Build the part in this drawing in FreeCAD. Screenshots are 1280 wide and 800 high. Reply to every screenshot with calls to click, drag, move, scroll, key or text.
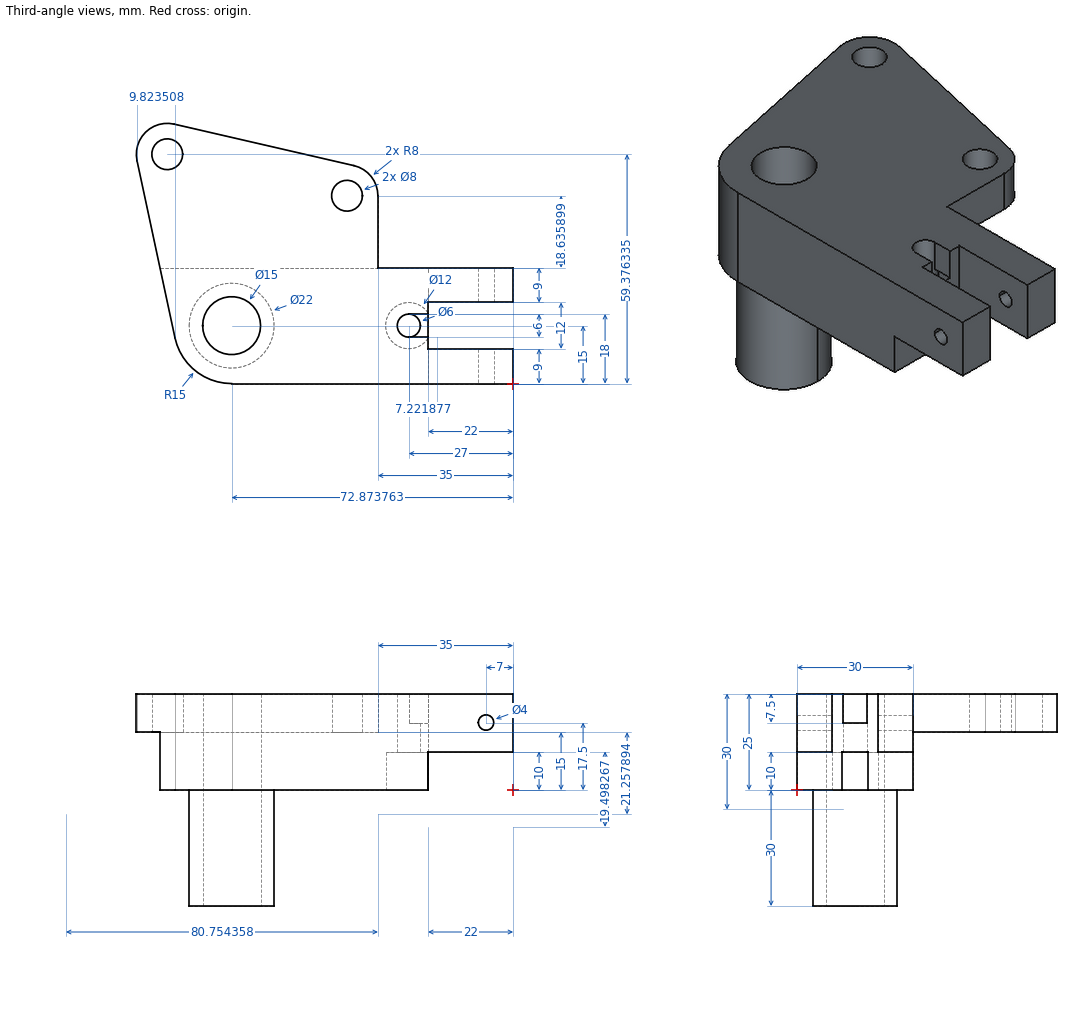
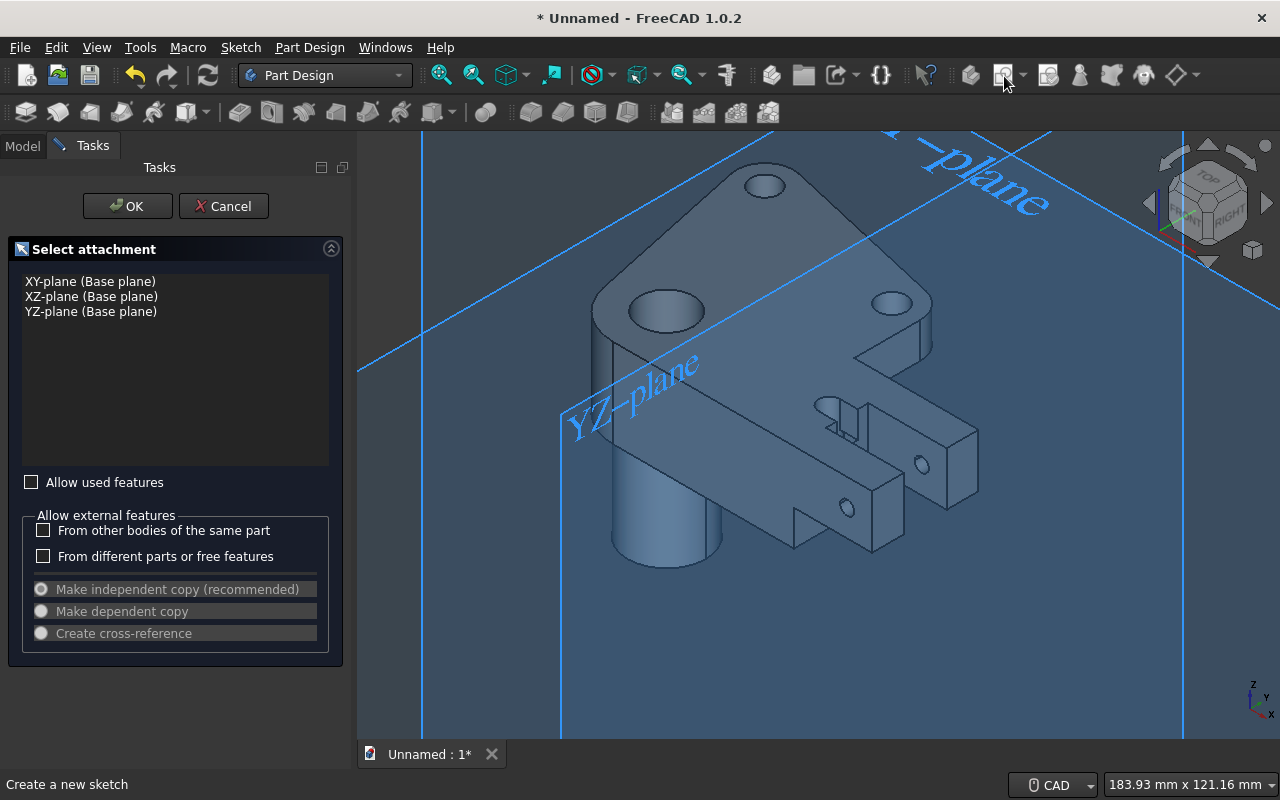
click(82, 282)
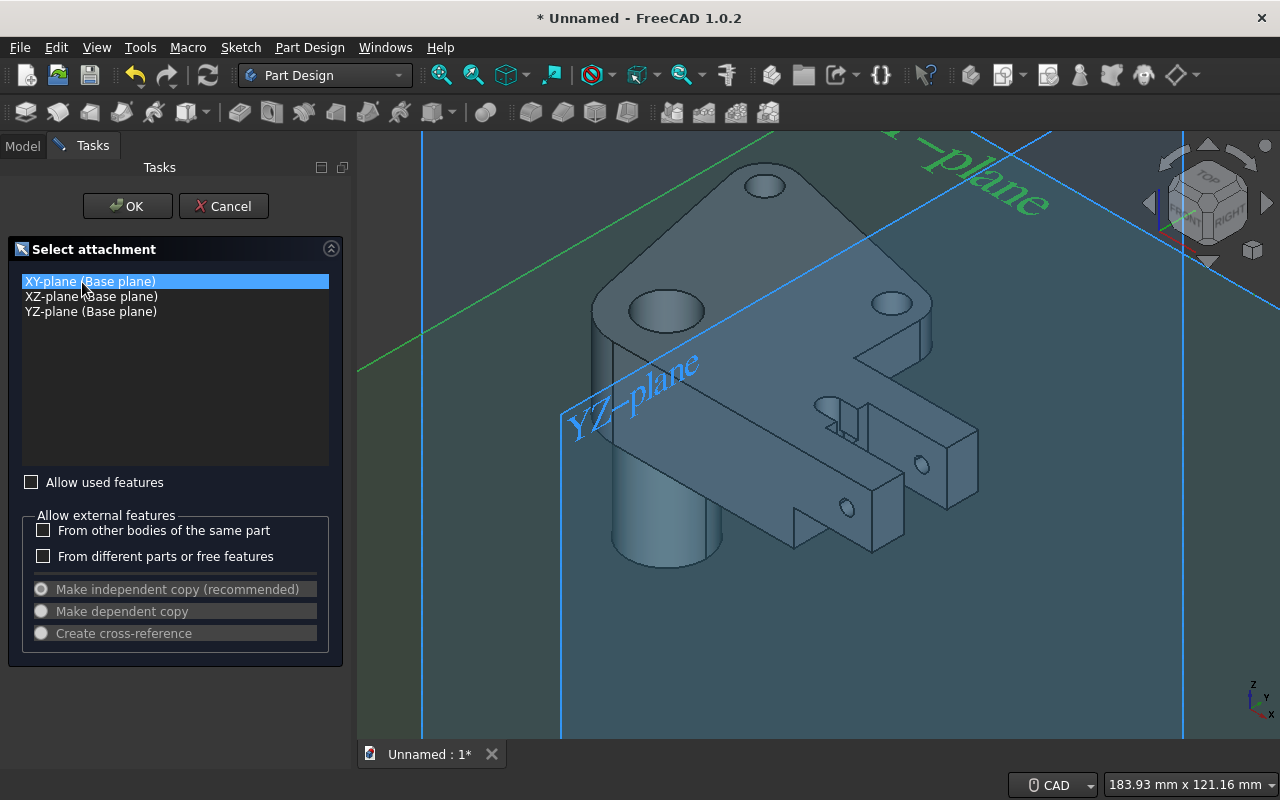
click(128, 206)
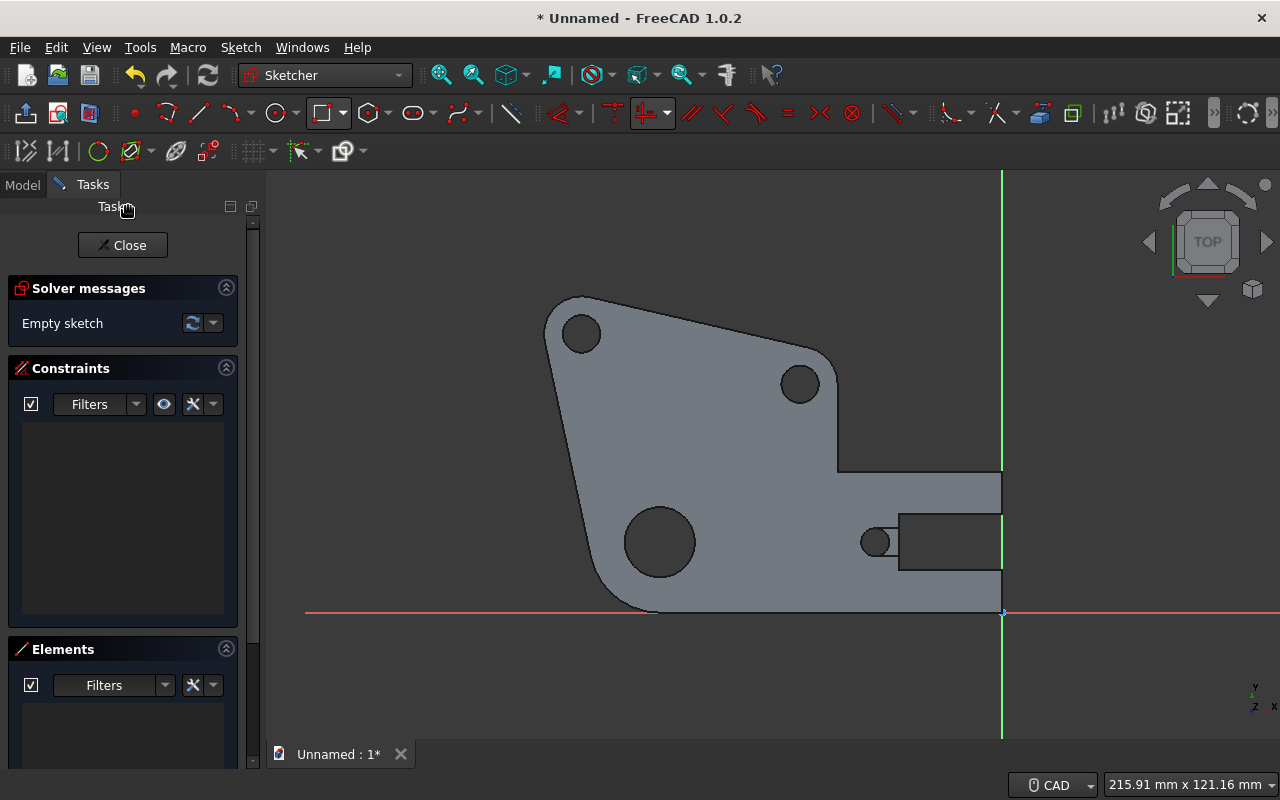
click(90, 114)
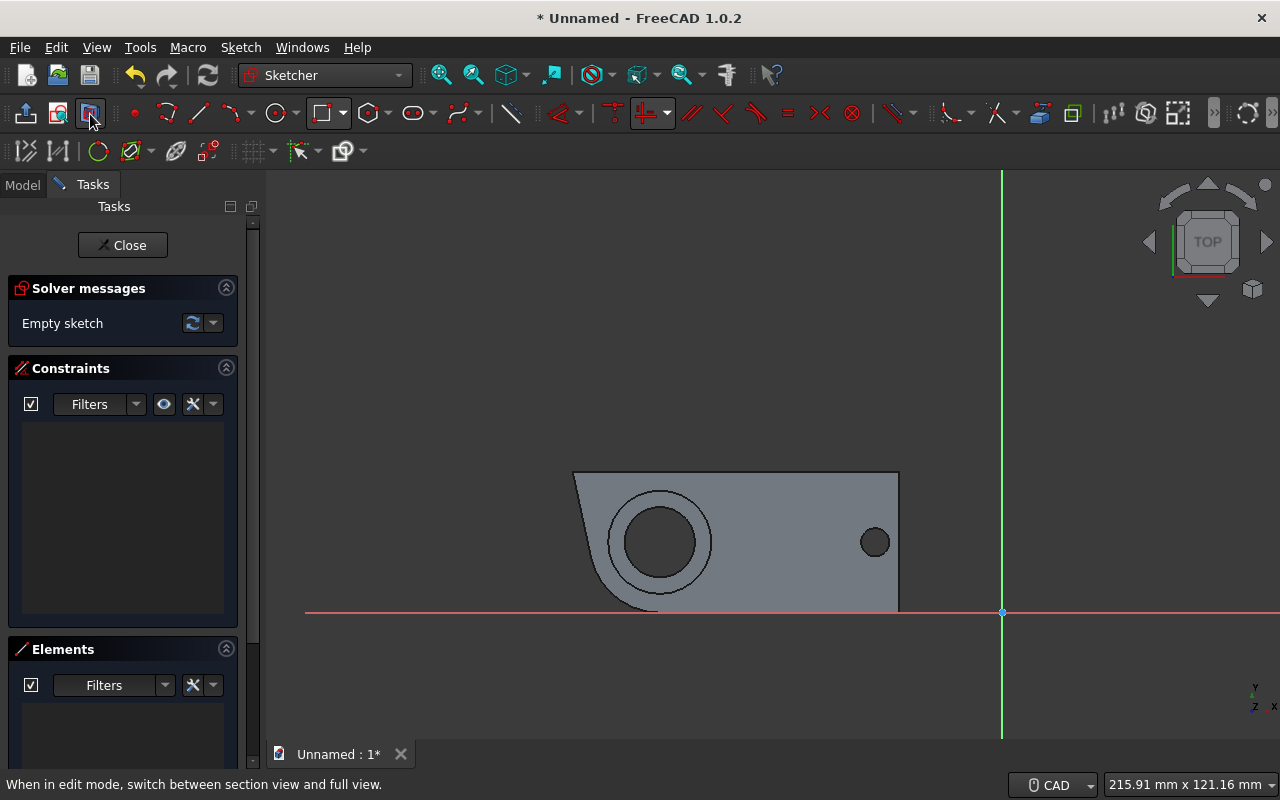
scroll(909, 560, up, 9)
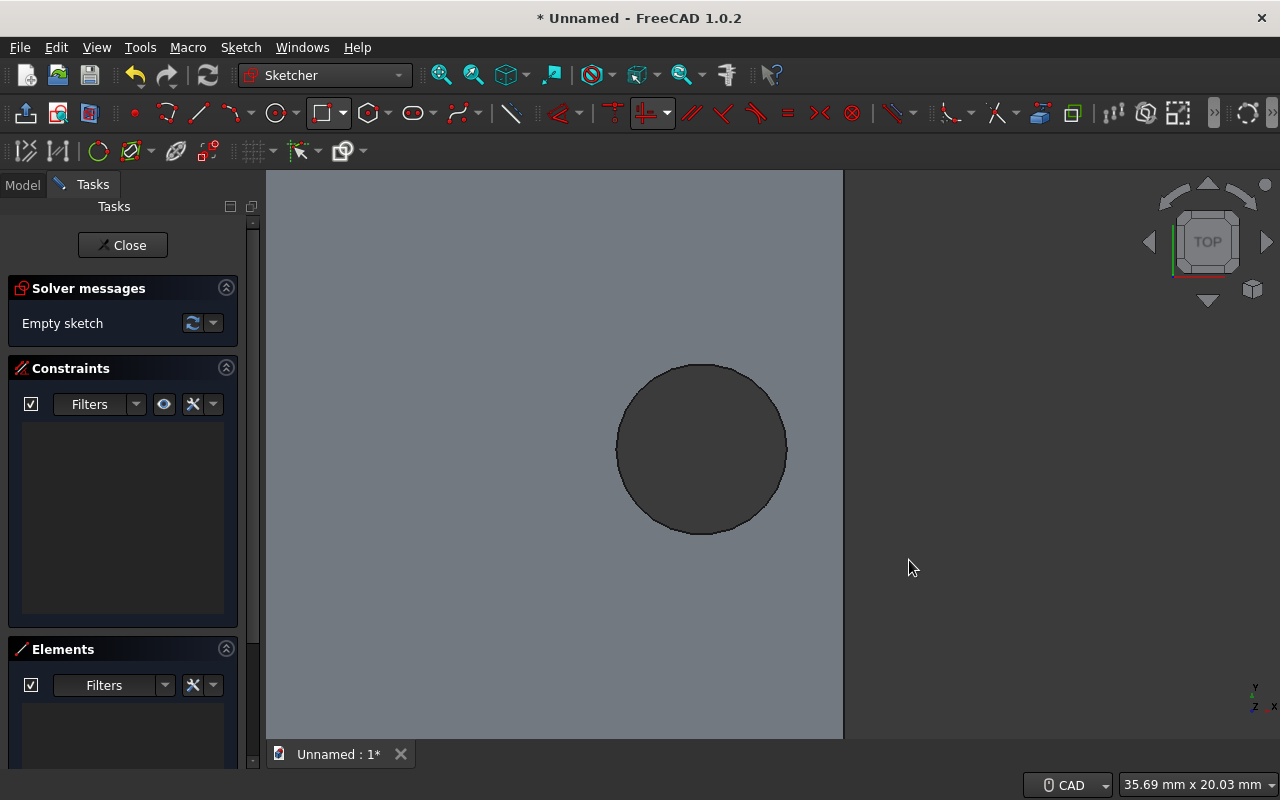
click(276, 114)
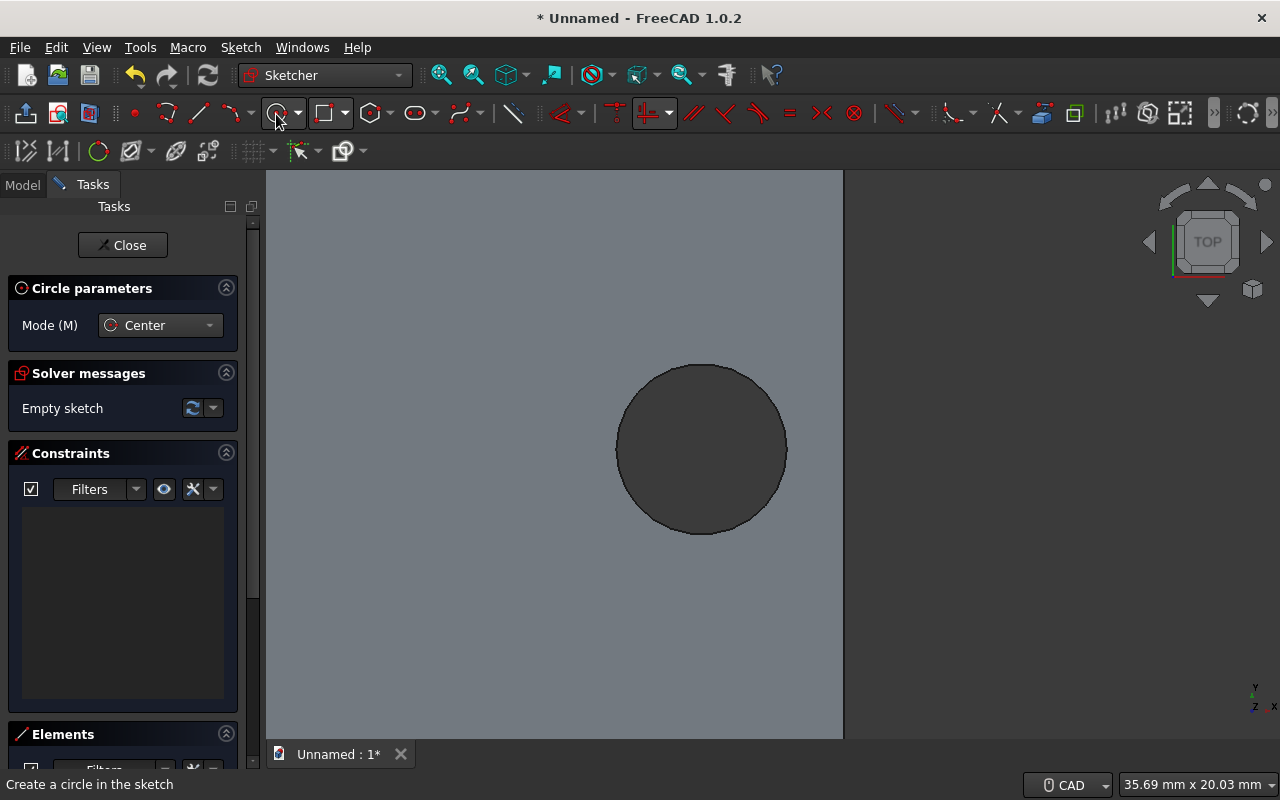
click(702, 449)
click(822, 329)
key(Escape)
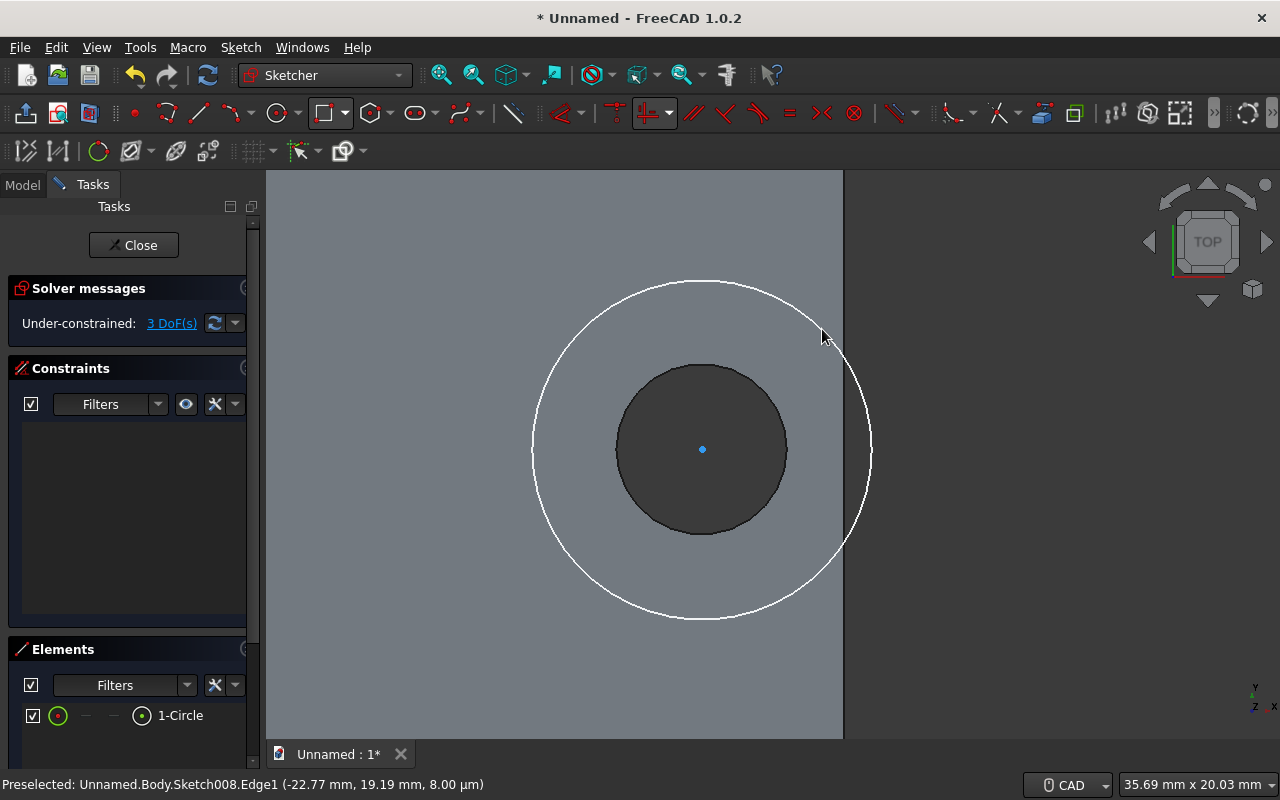
key(d)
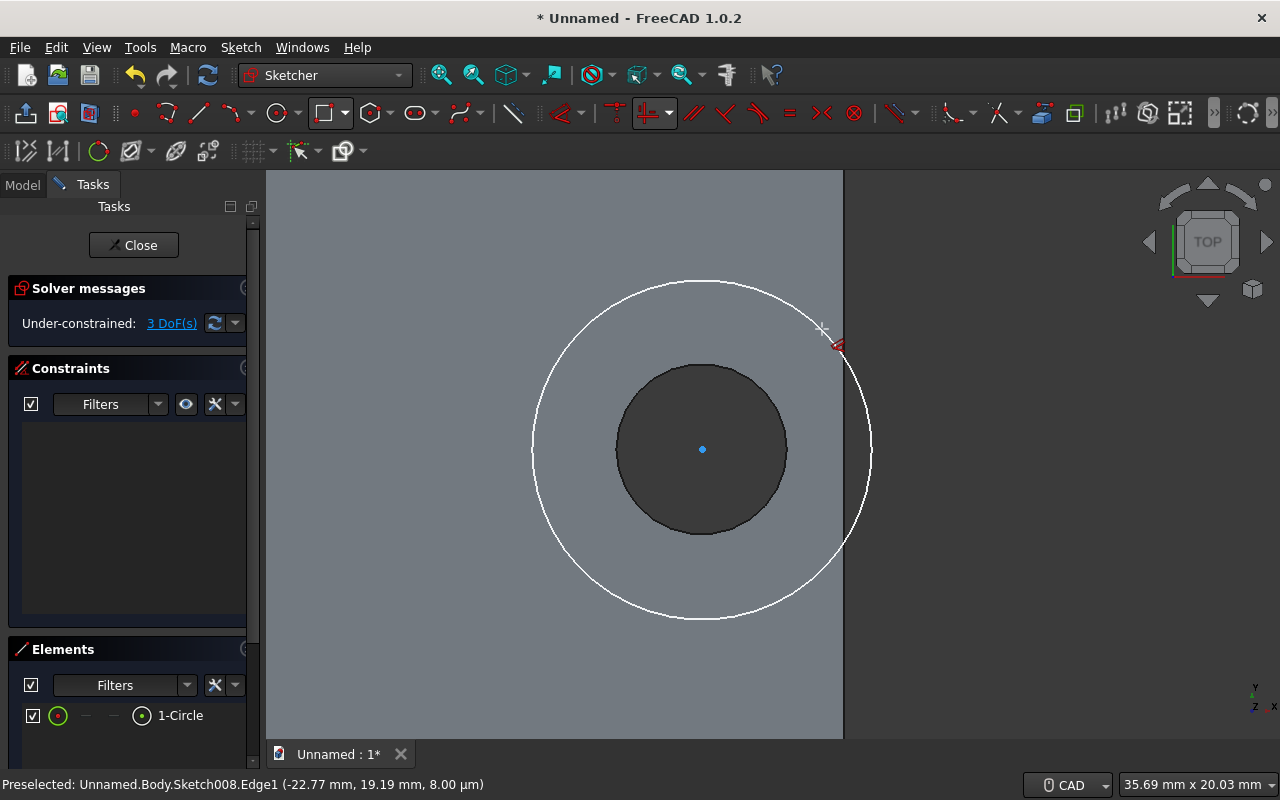
click(822, 330)
click(845, 307)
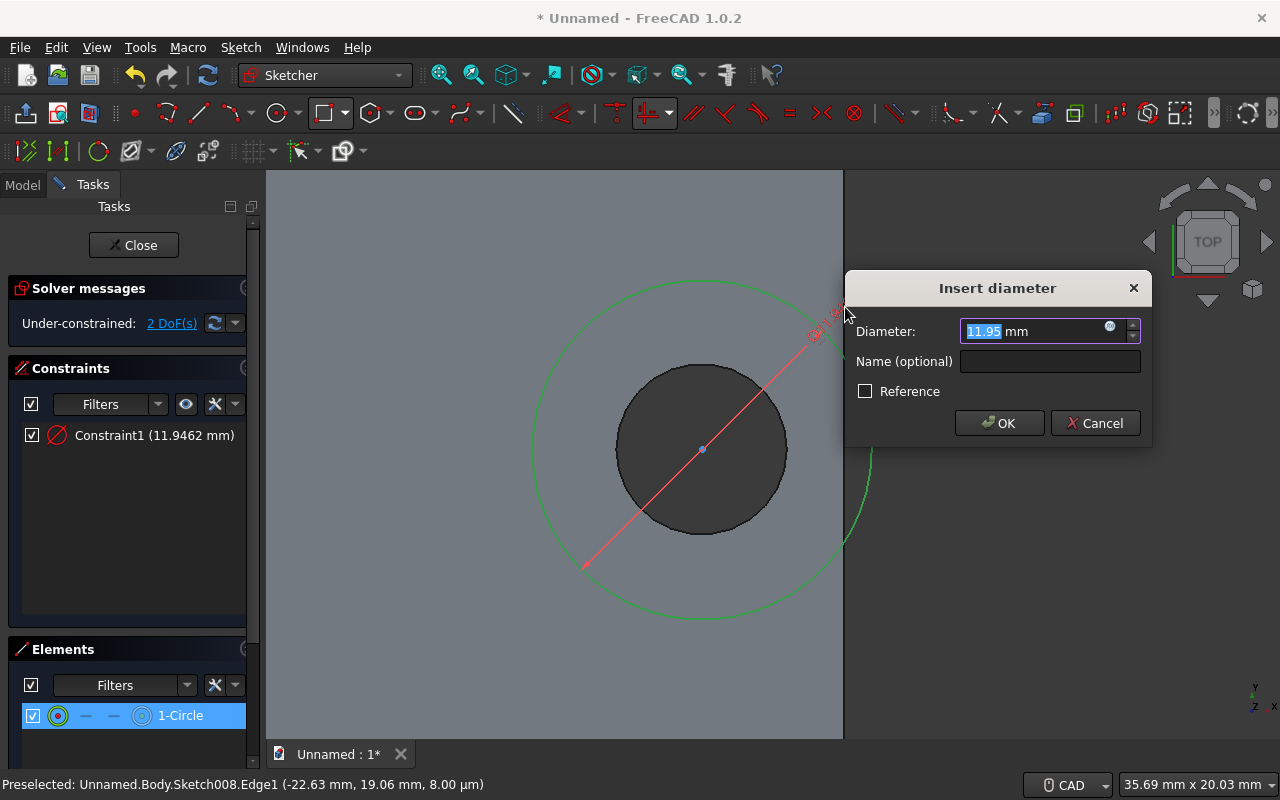
text(12)
key(Return)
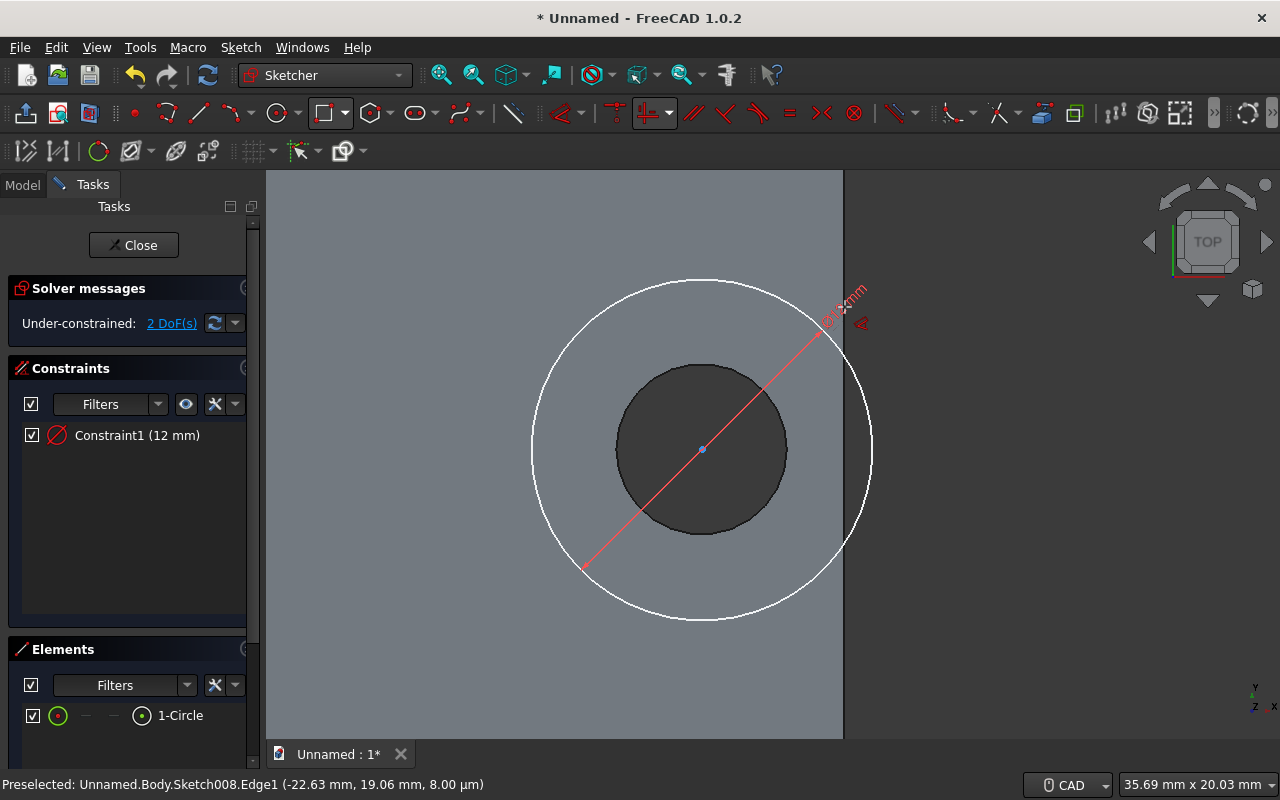
click(702, 450)
click(909, 416)